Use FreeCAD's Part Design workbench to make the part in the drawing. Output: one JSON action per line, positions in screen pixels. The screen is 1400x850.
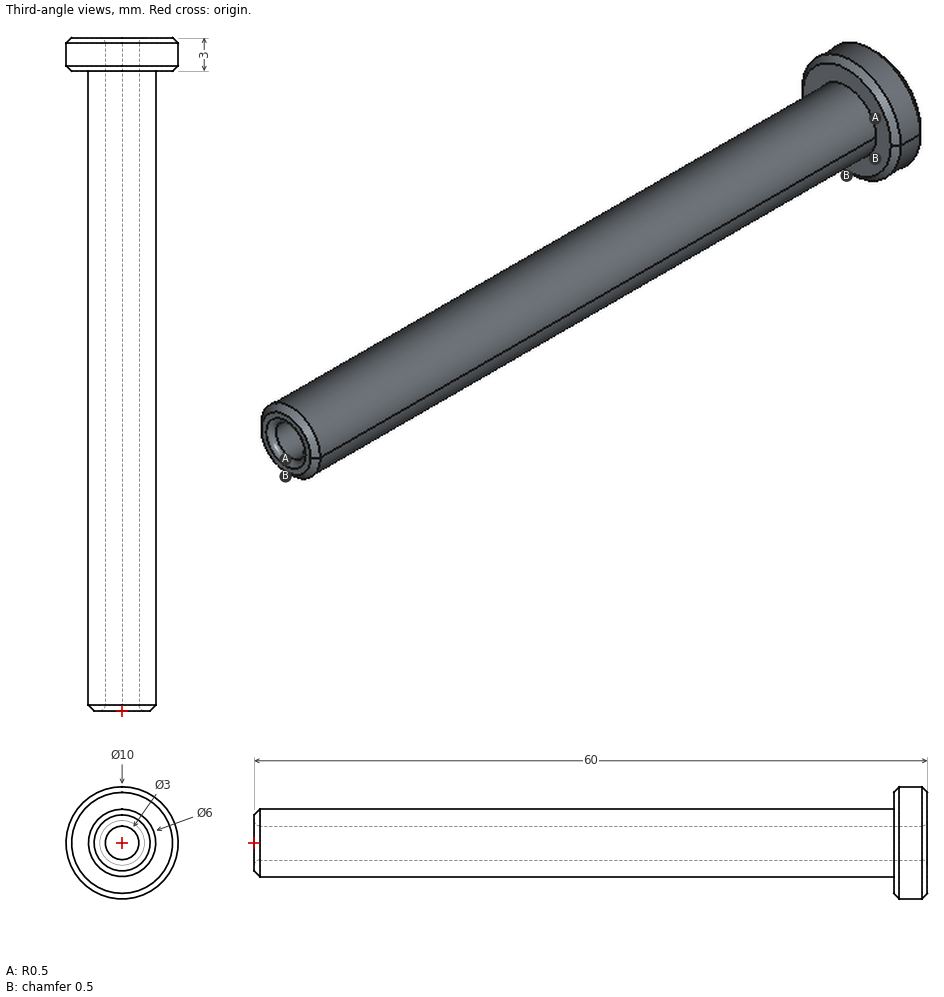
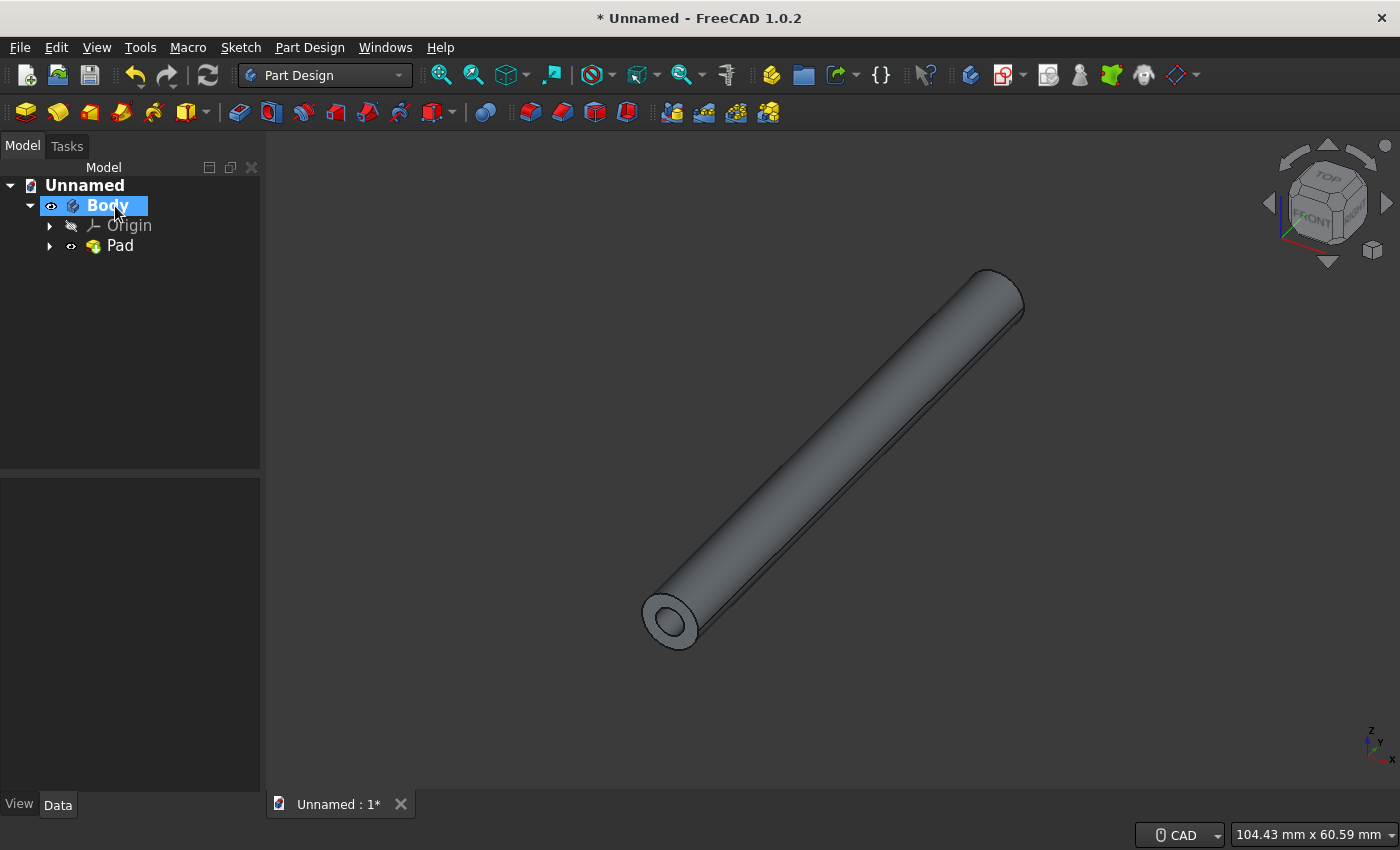
{"action": "left_click", "coordinate": [50, 226]}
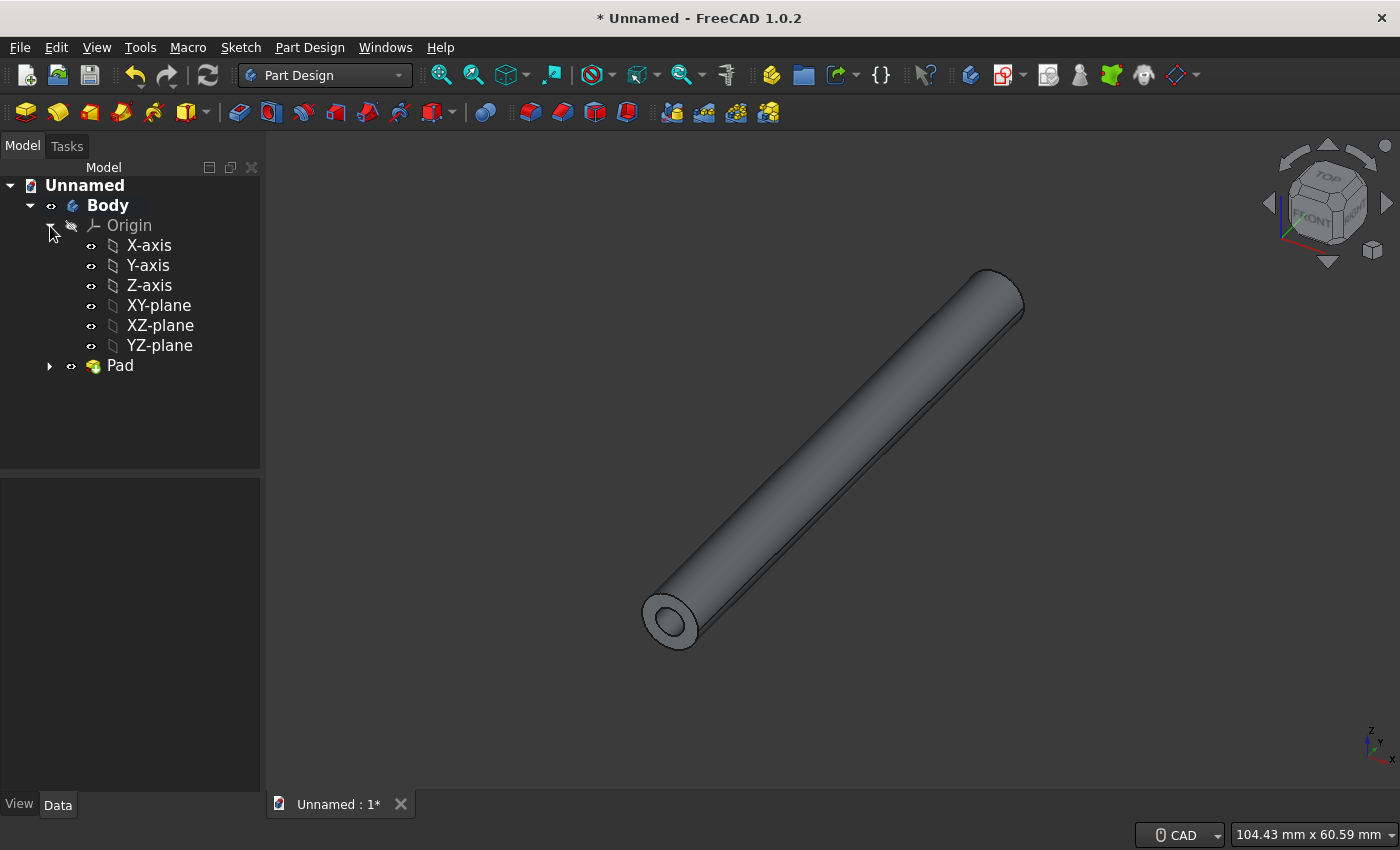
{"action": "left_click", "coordinate": [136, 326]}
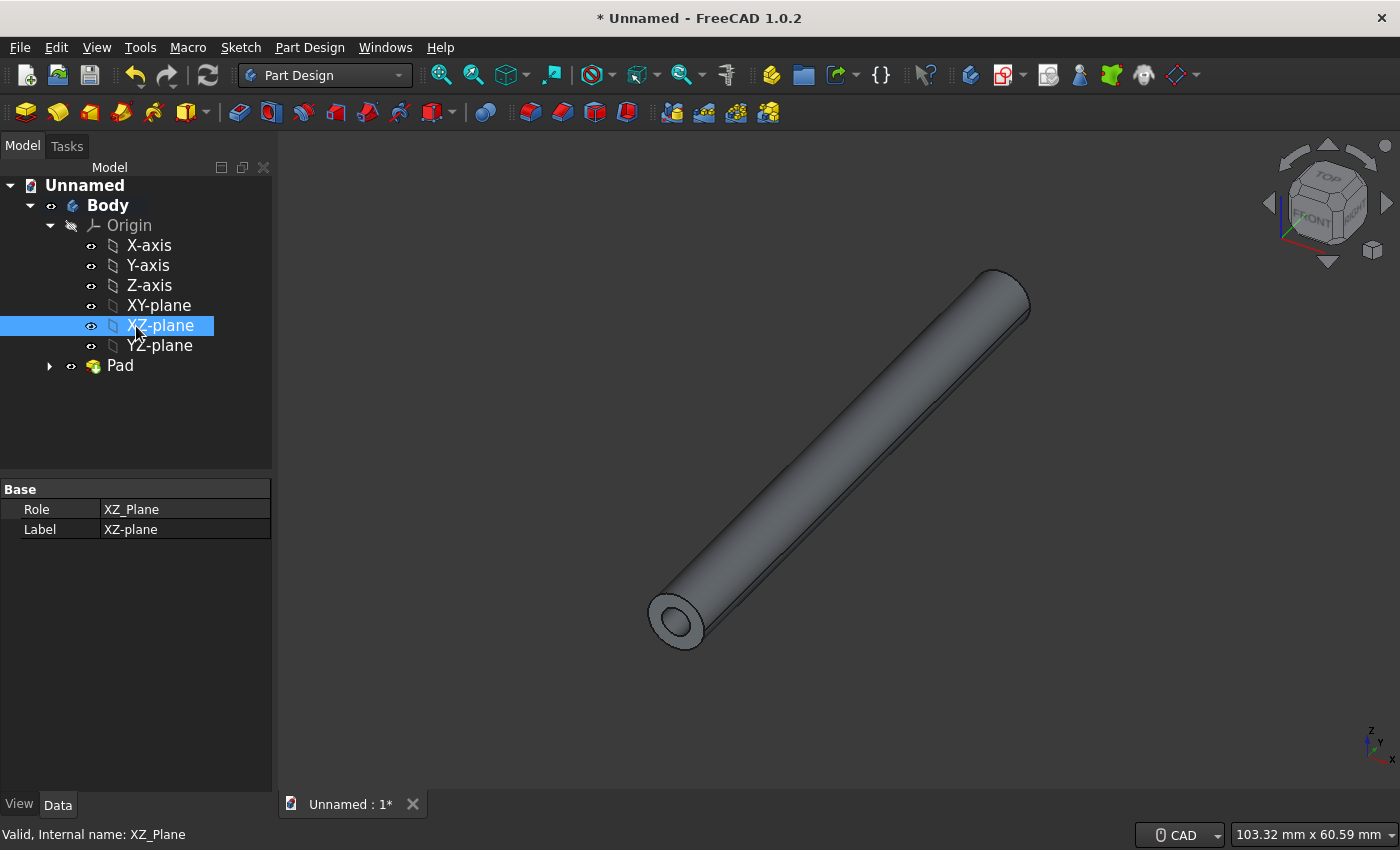
{"action": "left_click", "coordinate": [1176, 76]}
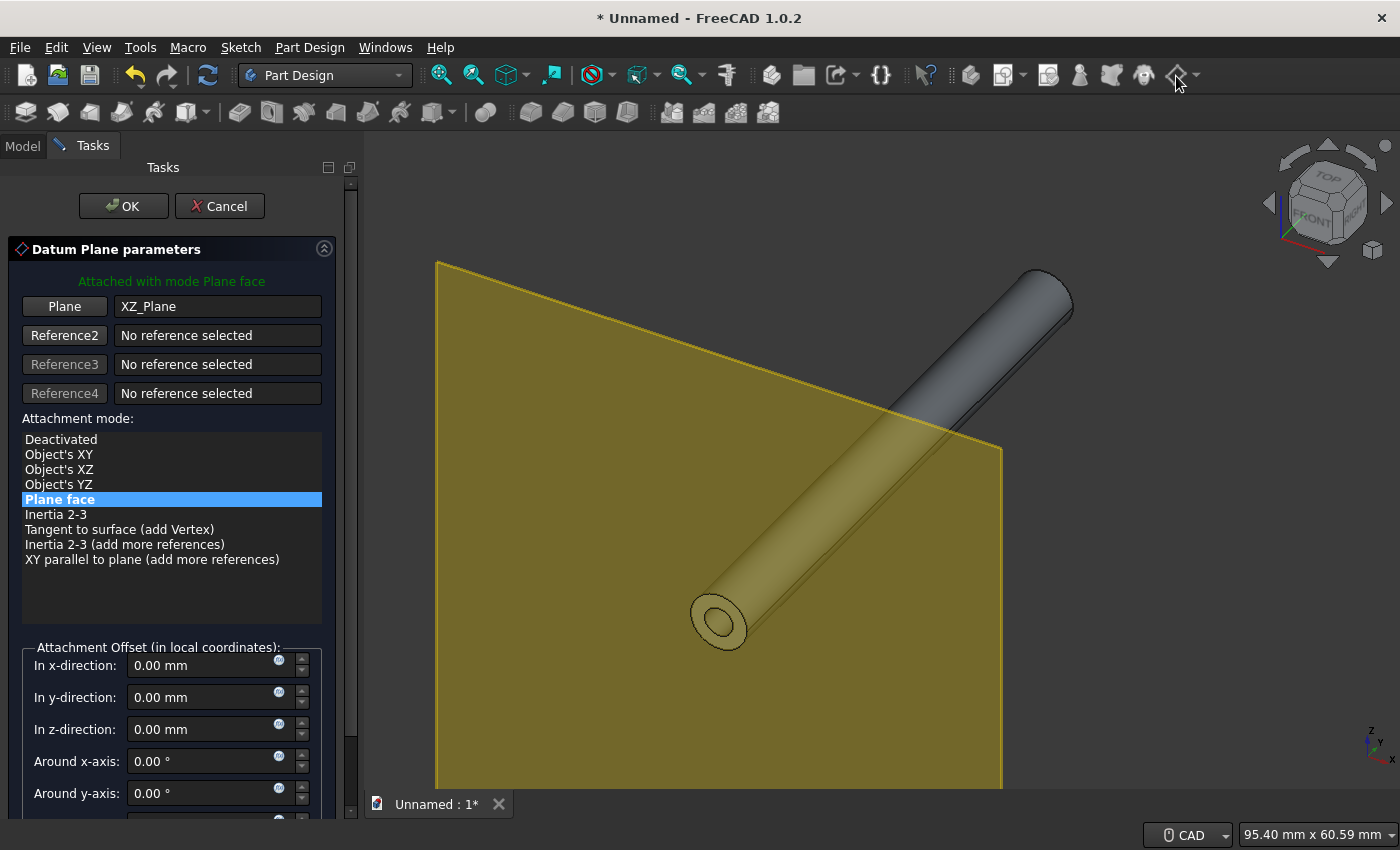
{"action": "triple_click", "coordinate": [210, 729]}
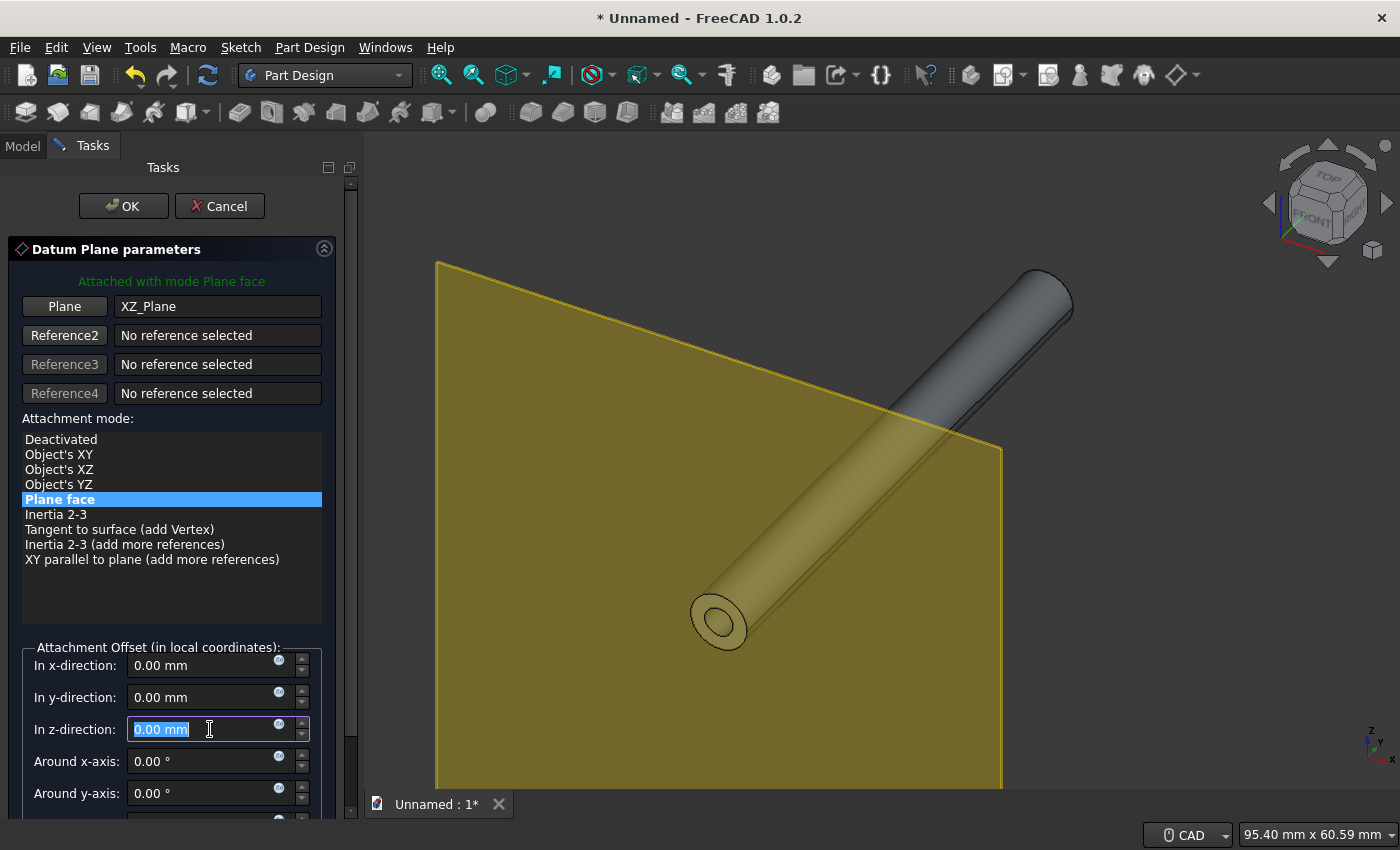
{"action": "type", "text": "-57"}
{"action": "key", "text": "Tab"}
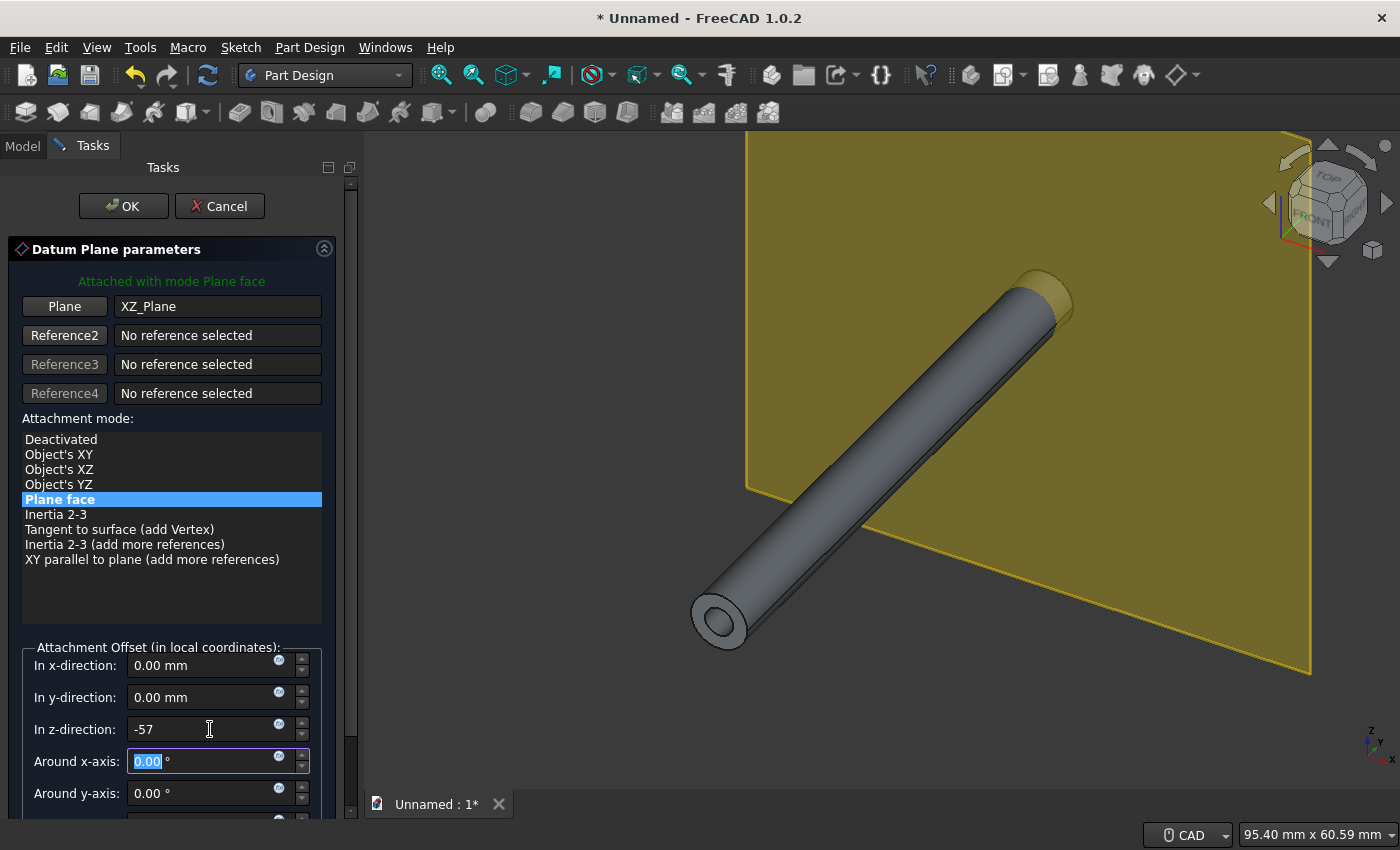
{"action": "left_click", "coordinate": [124, 206]}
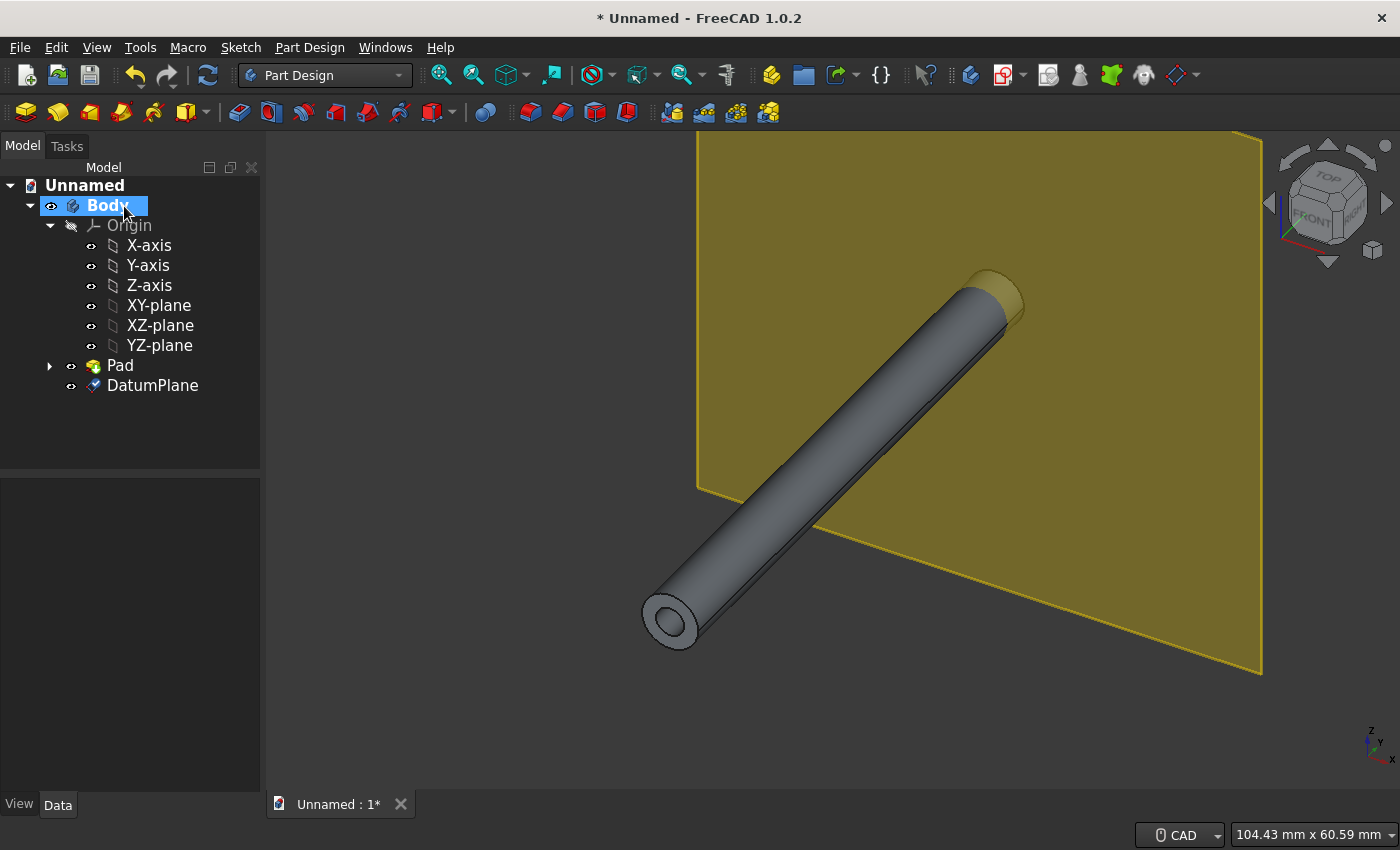
{"action": "left_click", "coordinate": [116, 386]}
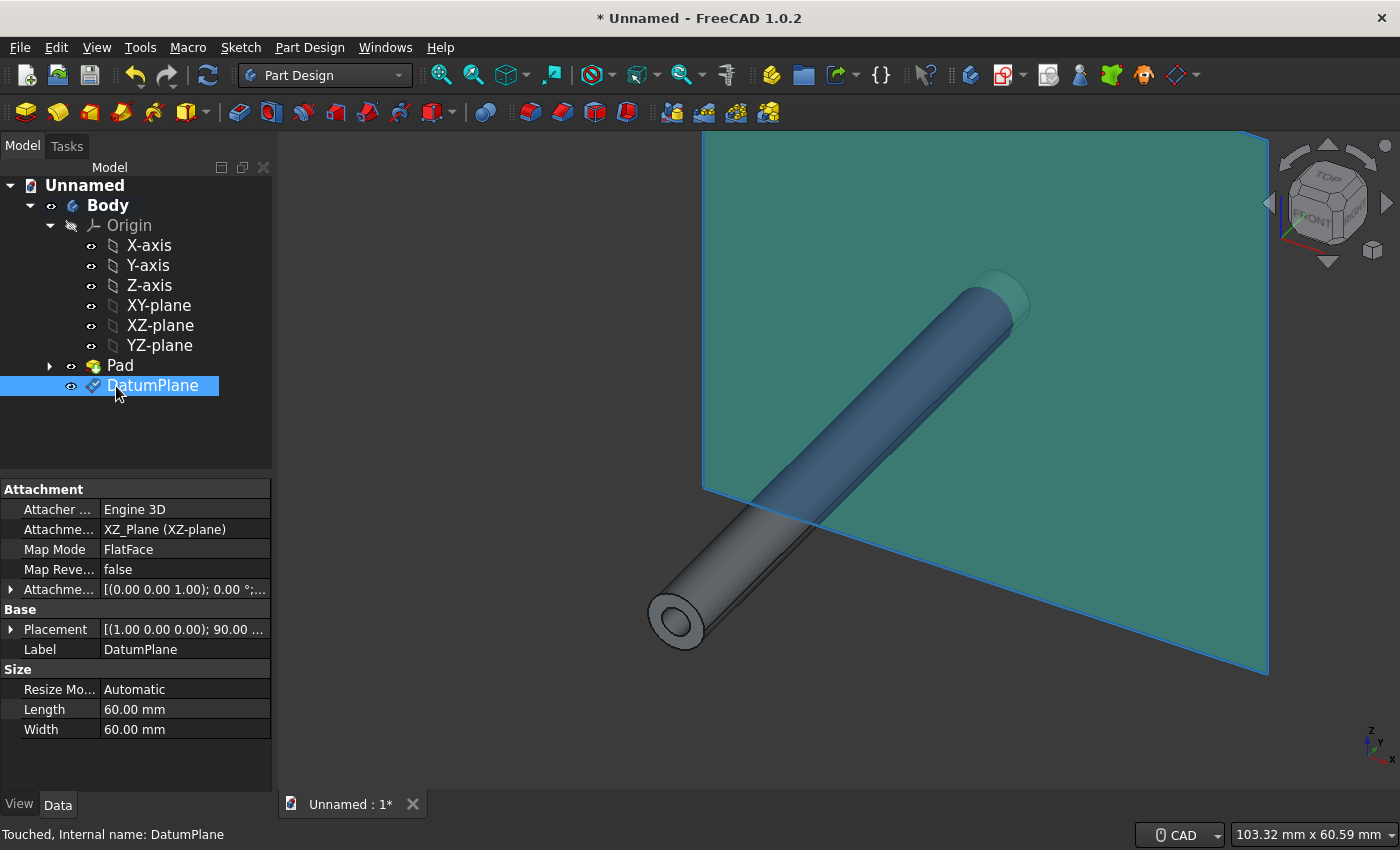
{"action": "left_click", "coordinate": [1004, 76]}